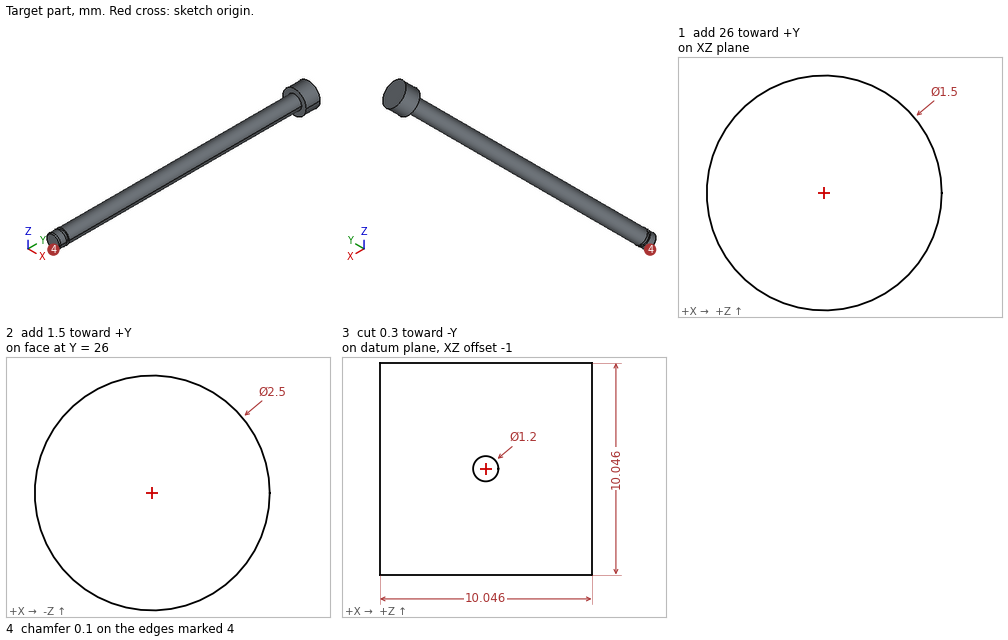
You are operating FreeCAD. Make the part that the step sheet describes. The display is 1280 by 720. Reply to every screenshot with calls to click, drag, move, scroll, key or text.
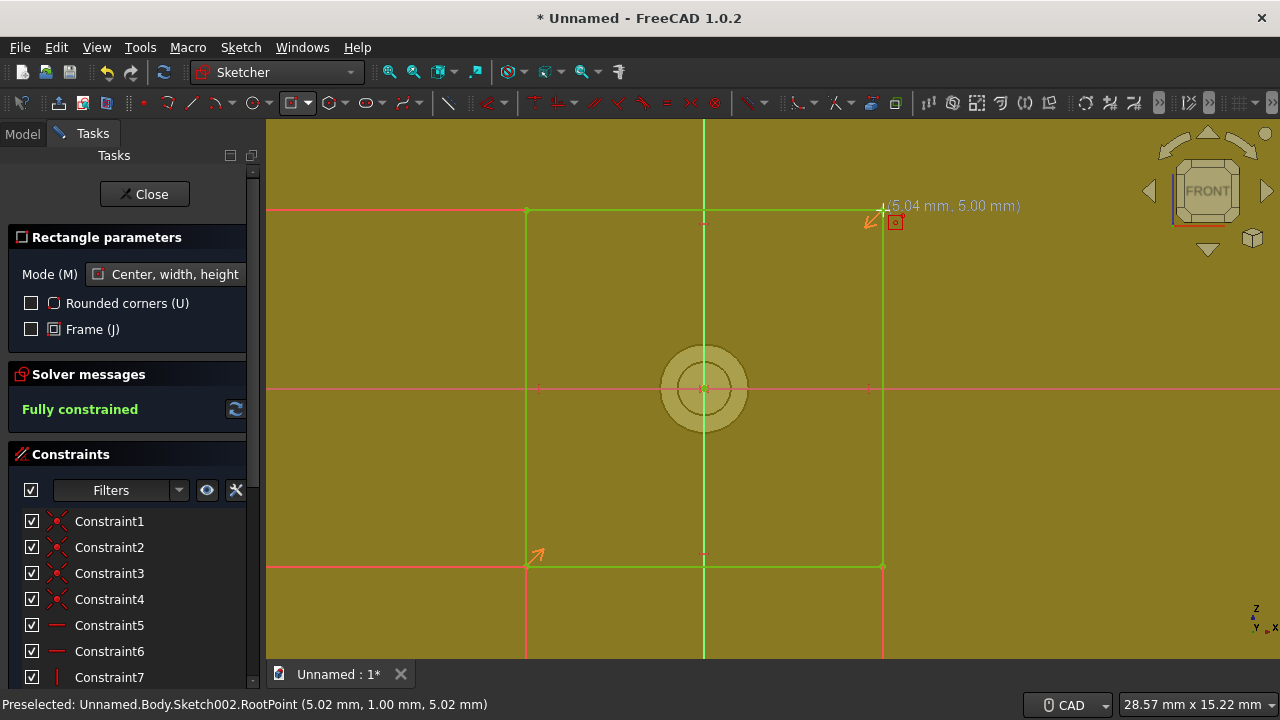
click(254, 104)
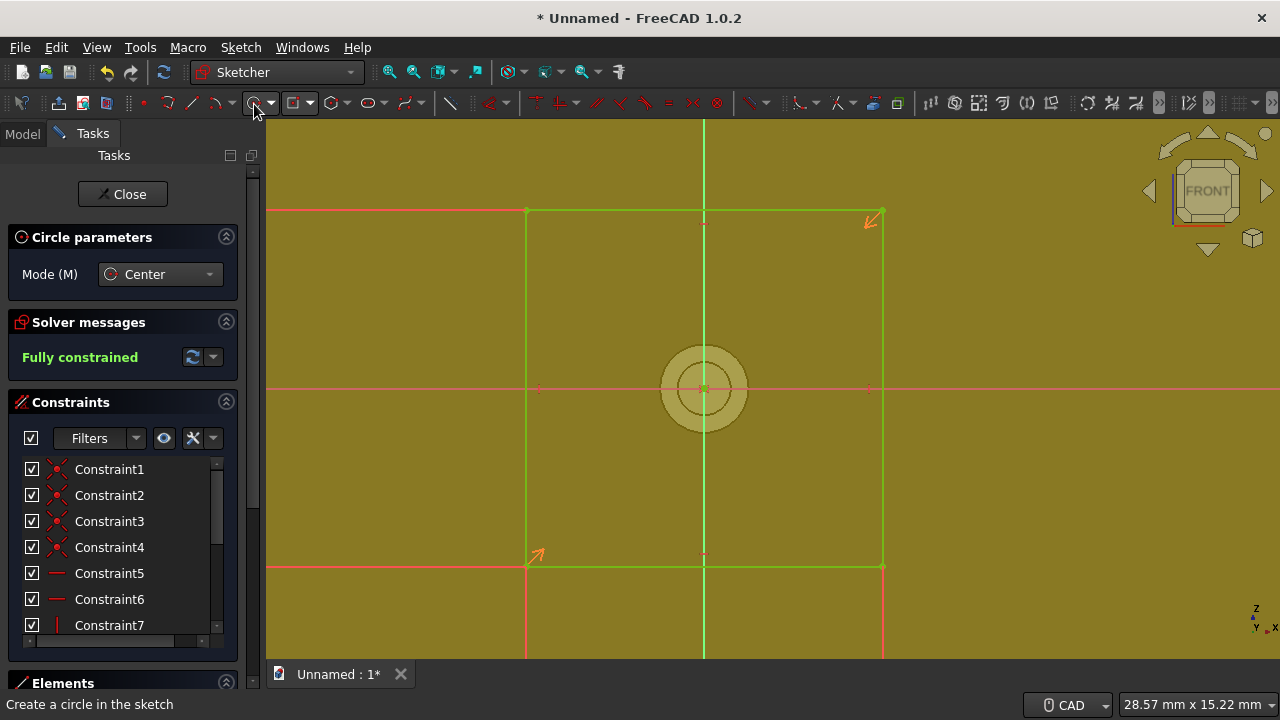
click(704, 389)
move(719, 374)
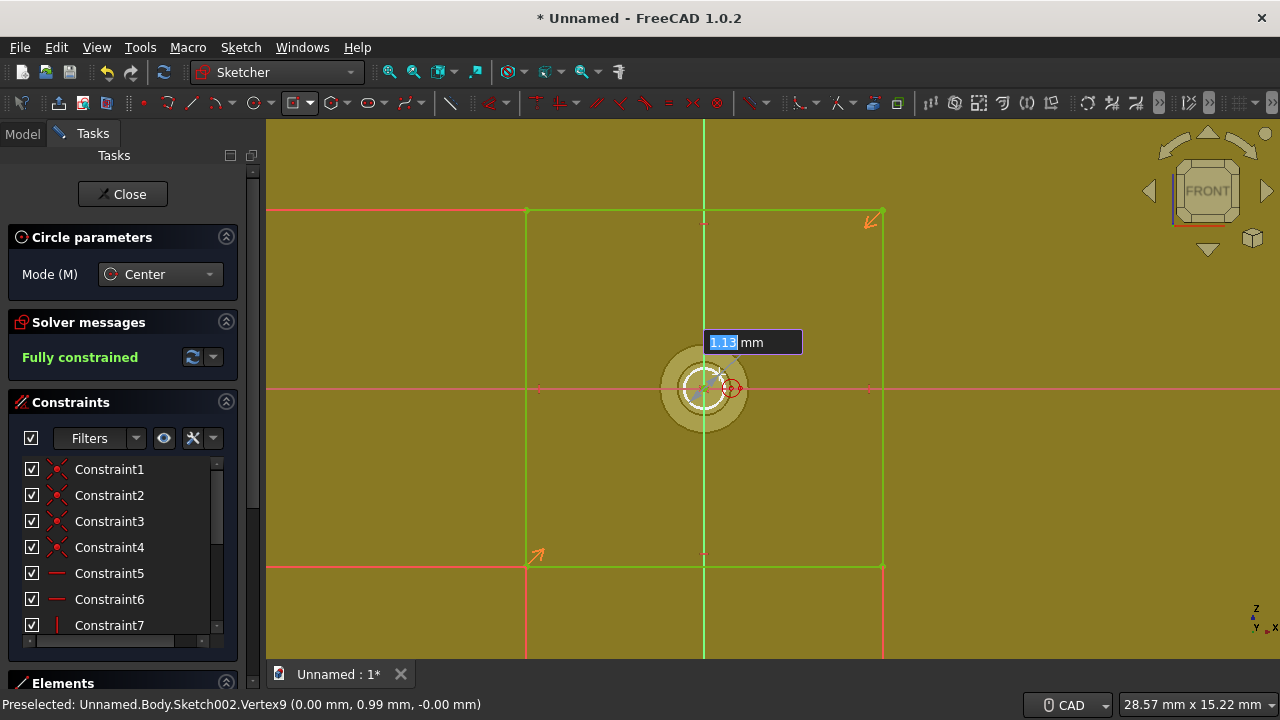
text(1.2)
key(Return)
key(Escape)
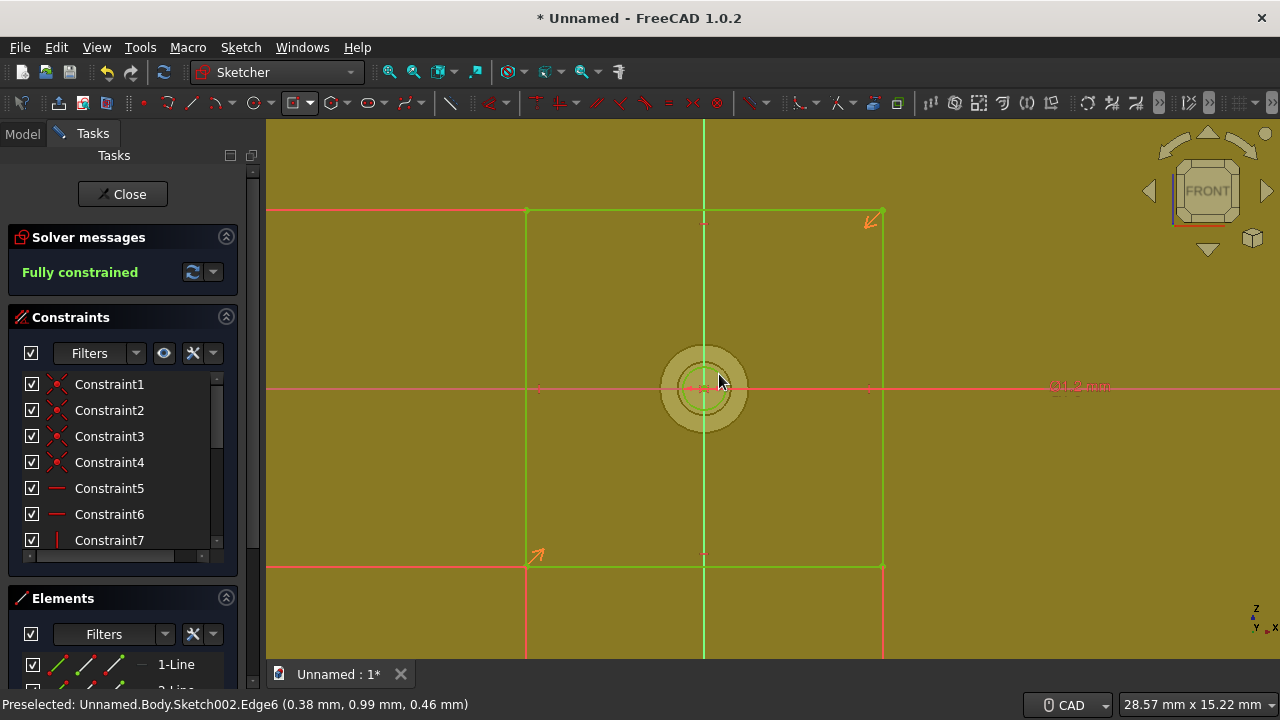
click(123, 194)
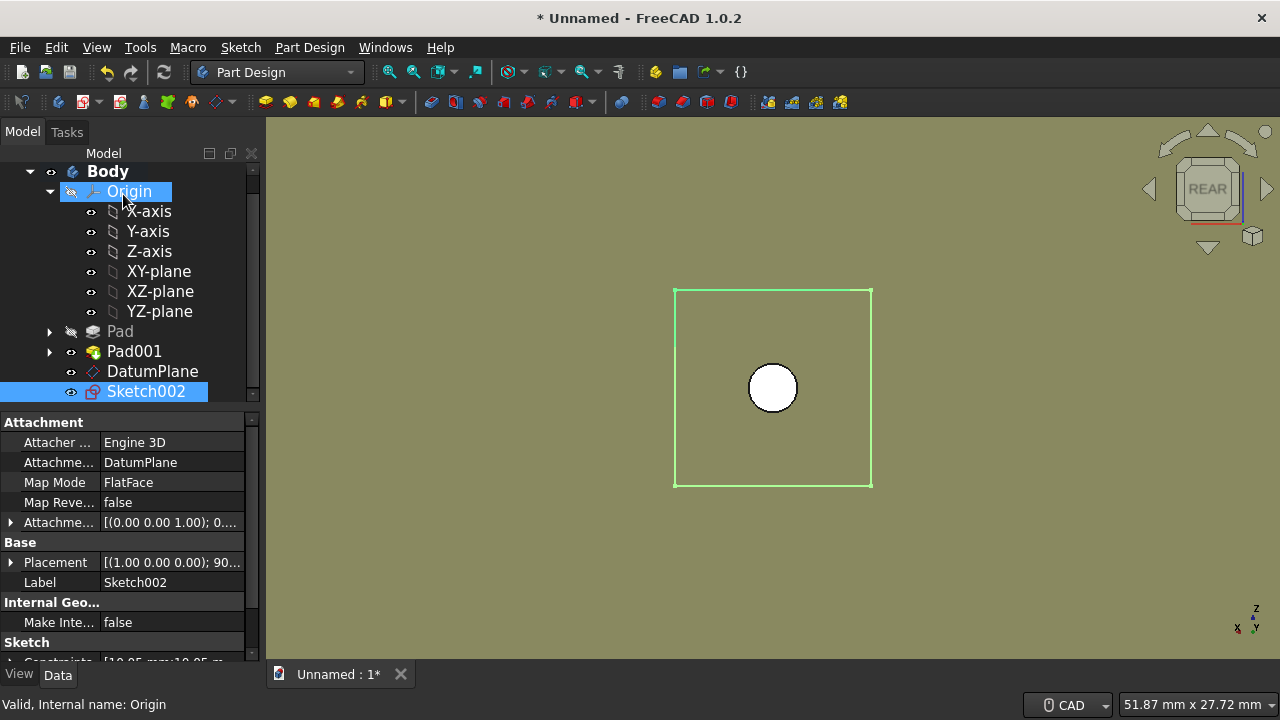
click(432, 102)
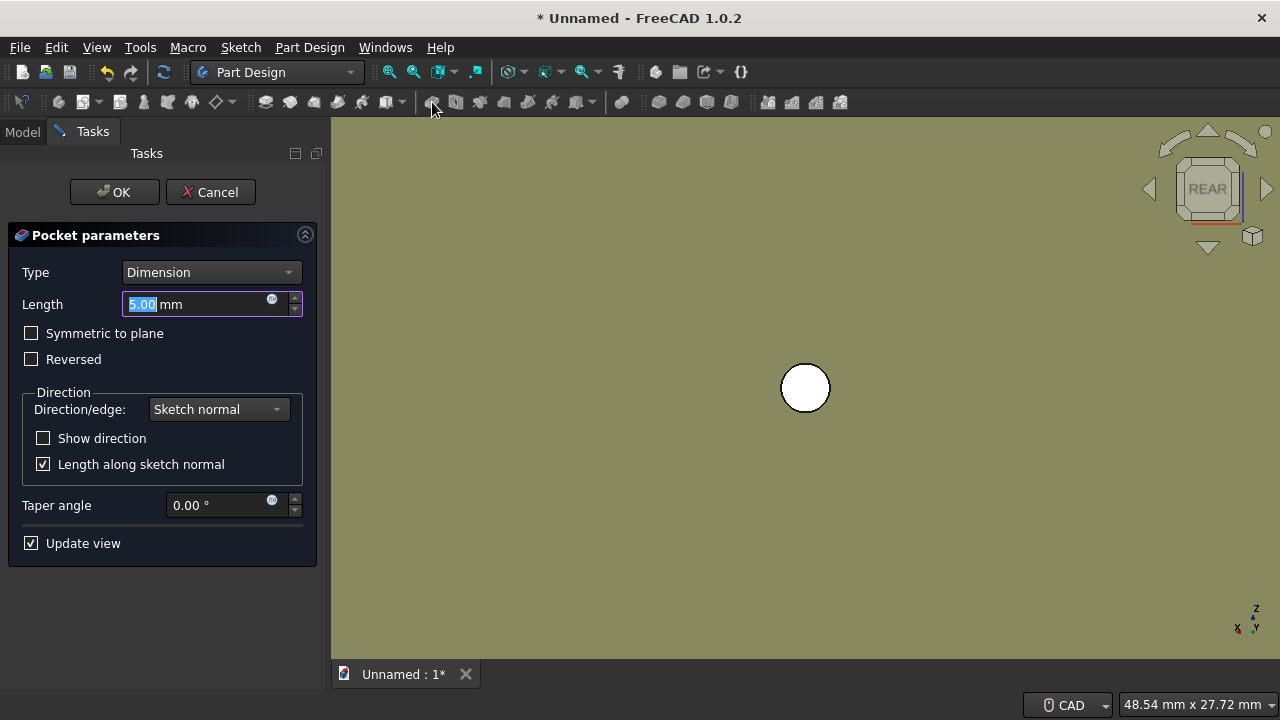
text(0.3)
key(Tab)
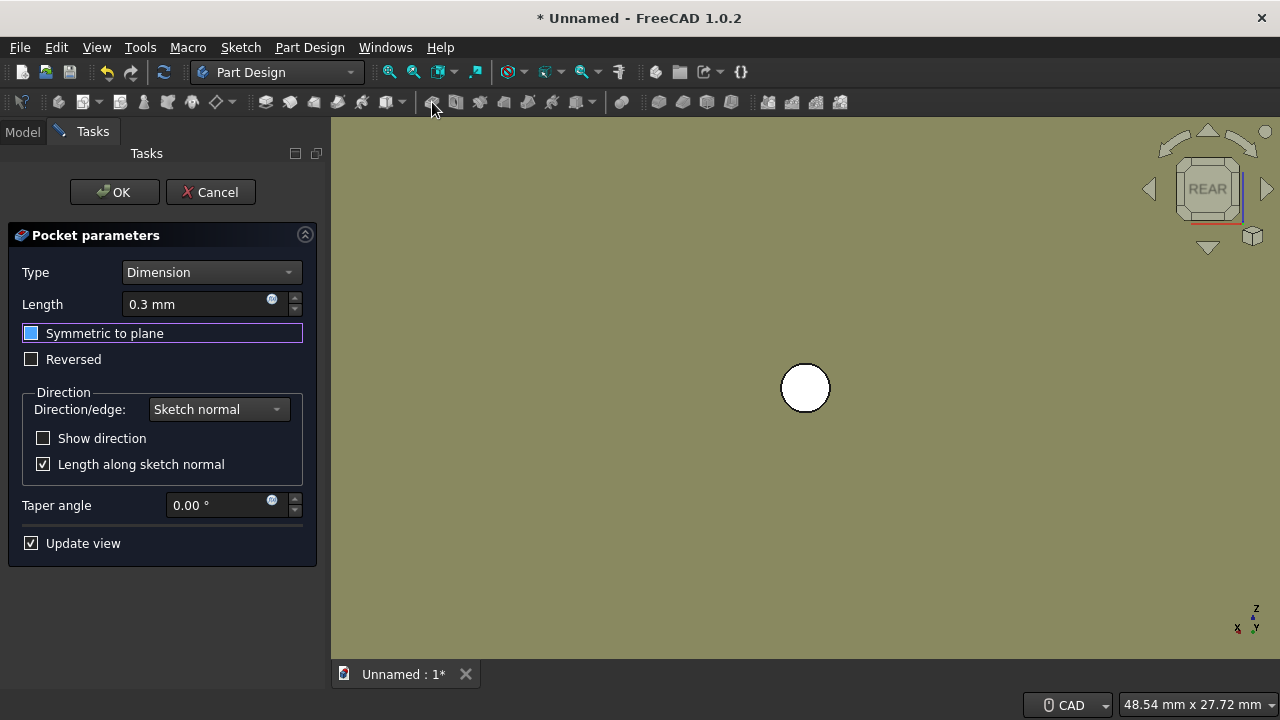
click(30, 359)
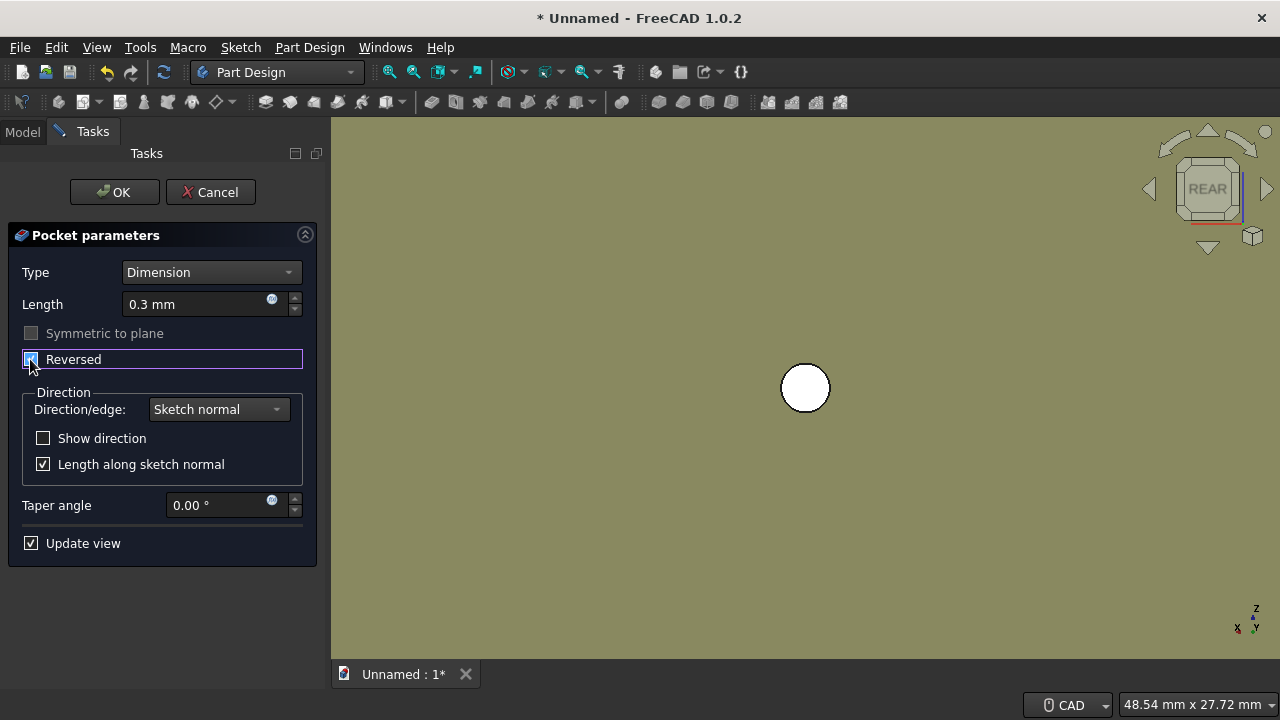
click(115, 192)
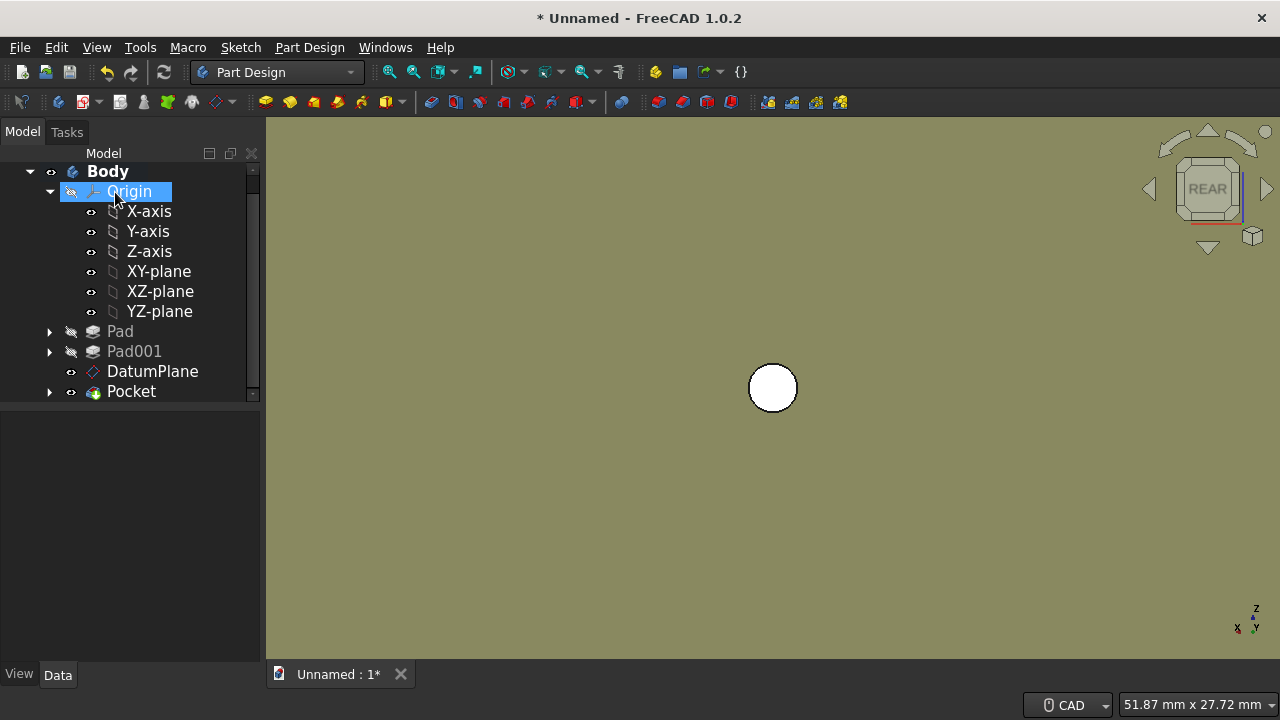
click(116, 372)
key(space)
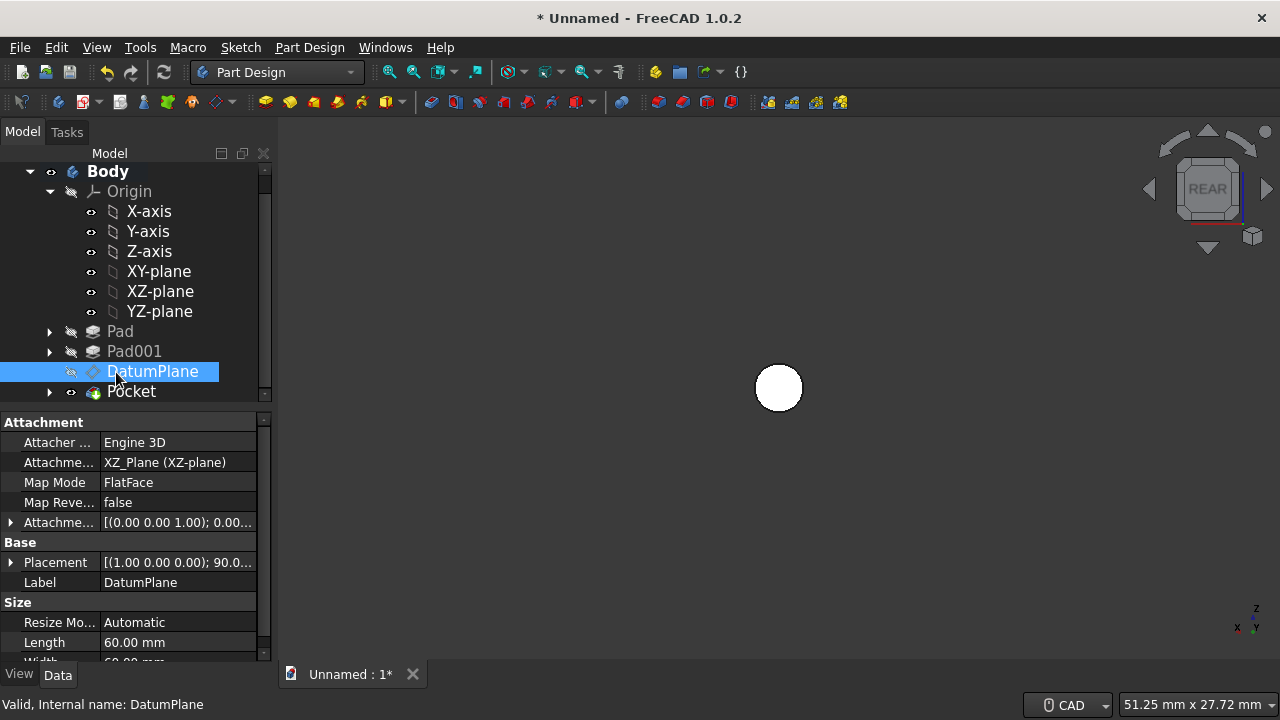
click(390, 72)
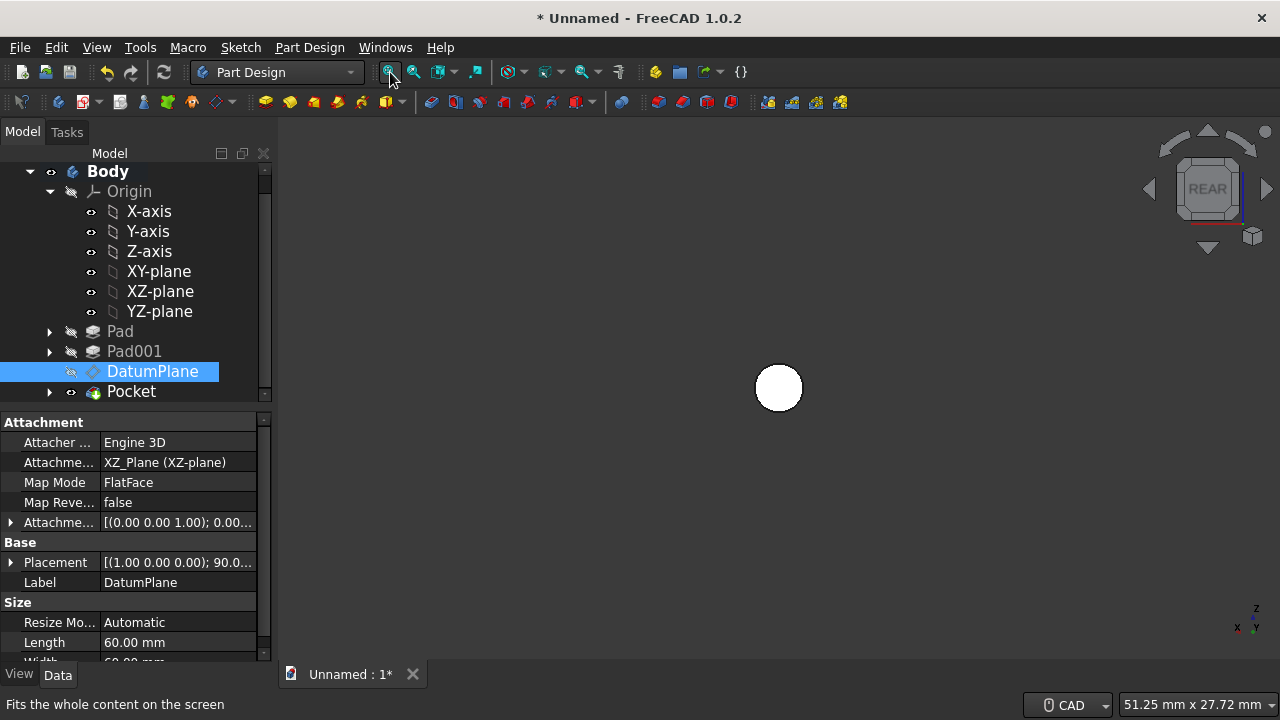
key(0)